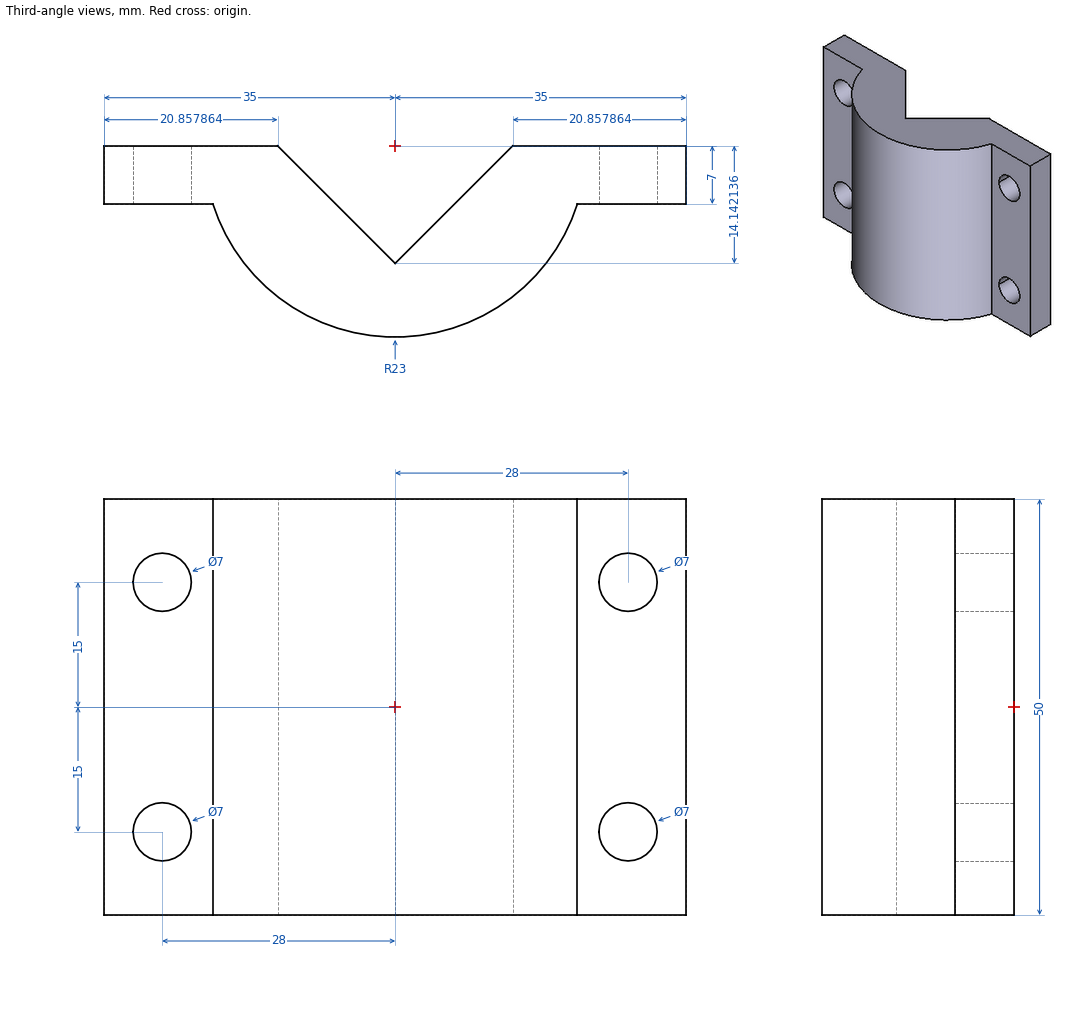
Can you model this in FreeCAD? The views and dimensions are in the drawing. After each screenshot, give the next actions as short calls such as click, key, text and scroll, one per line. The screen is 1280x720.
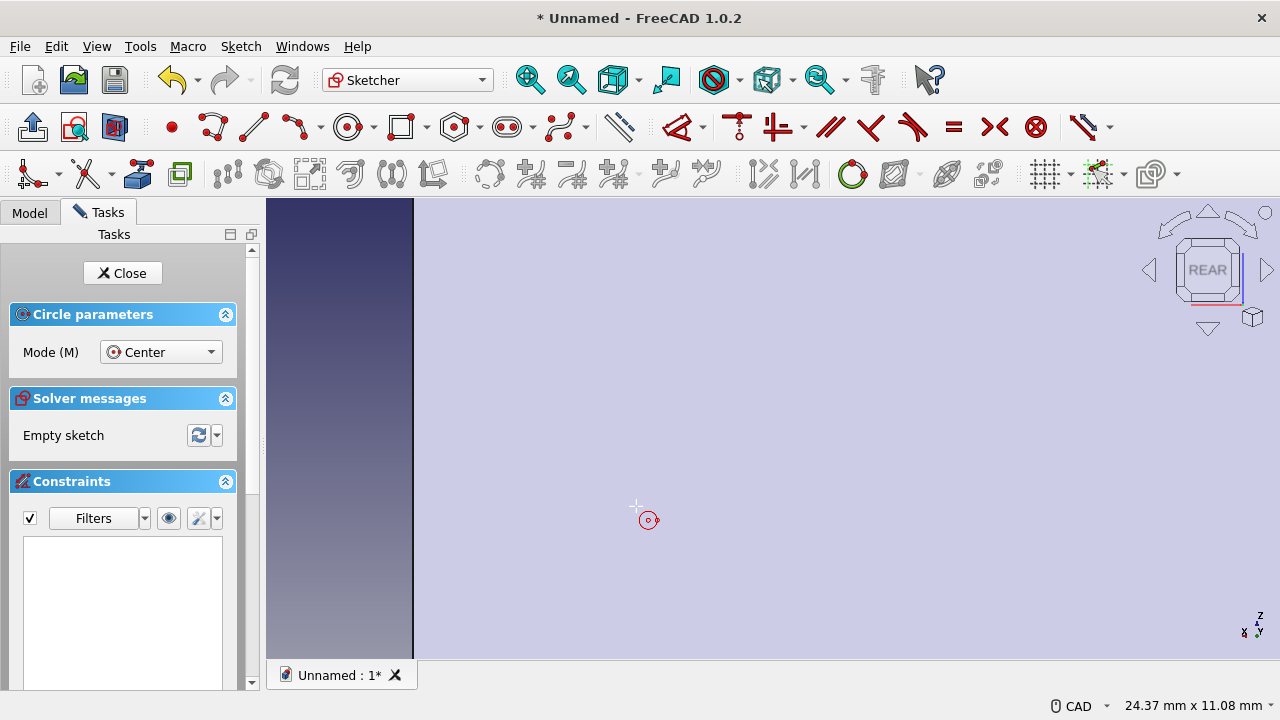
click(705, 425)
click(808, 322)
key(Escape)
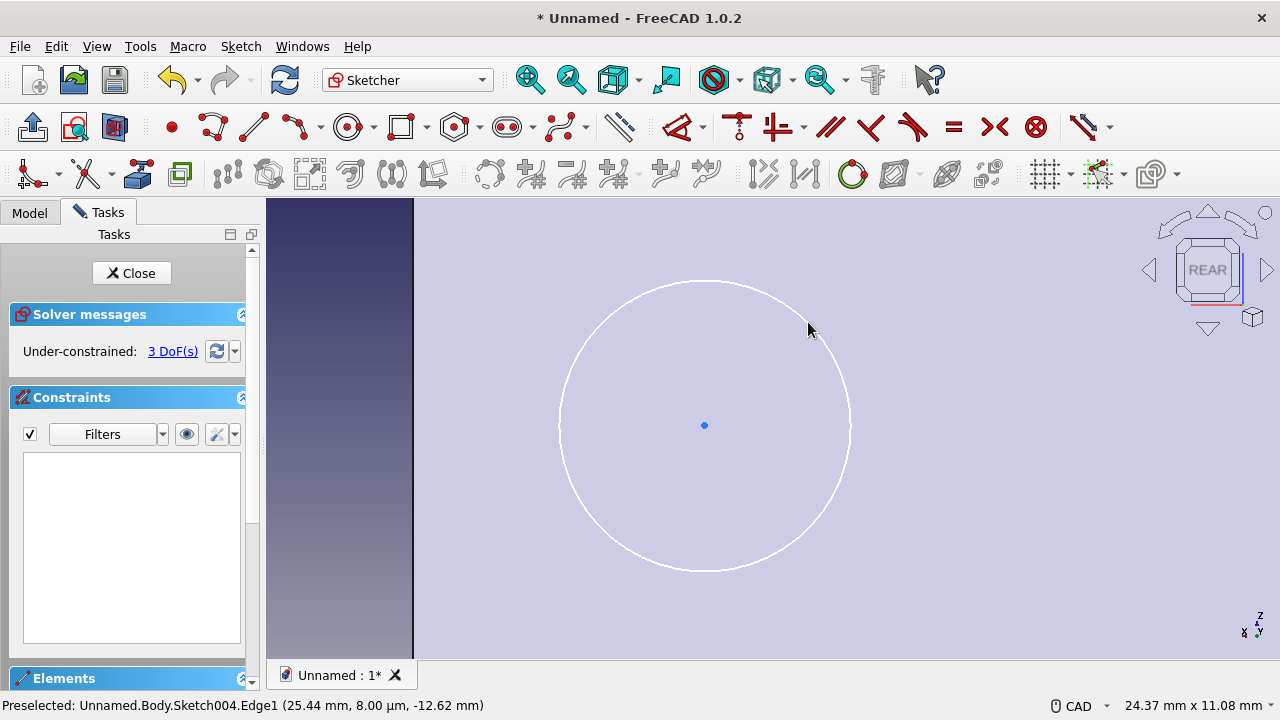
key(d)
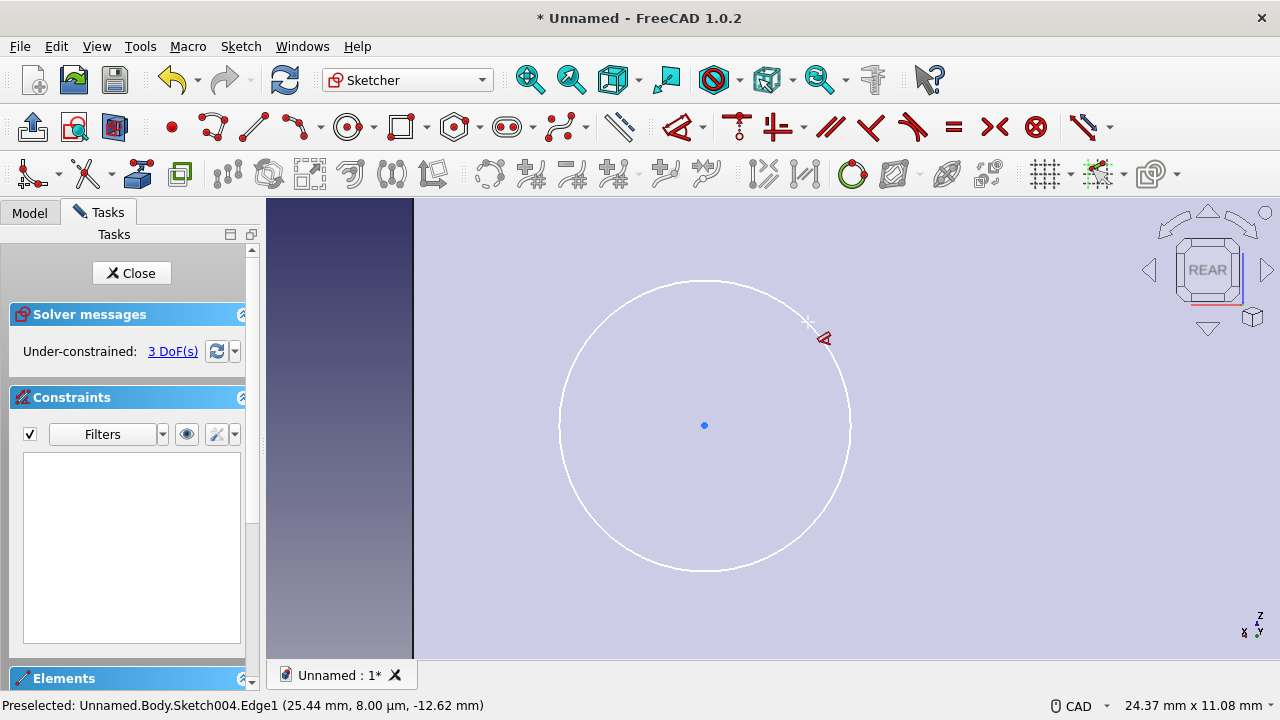
click(808, 323)
click(831, 300)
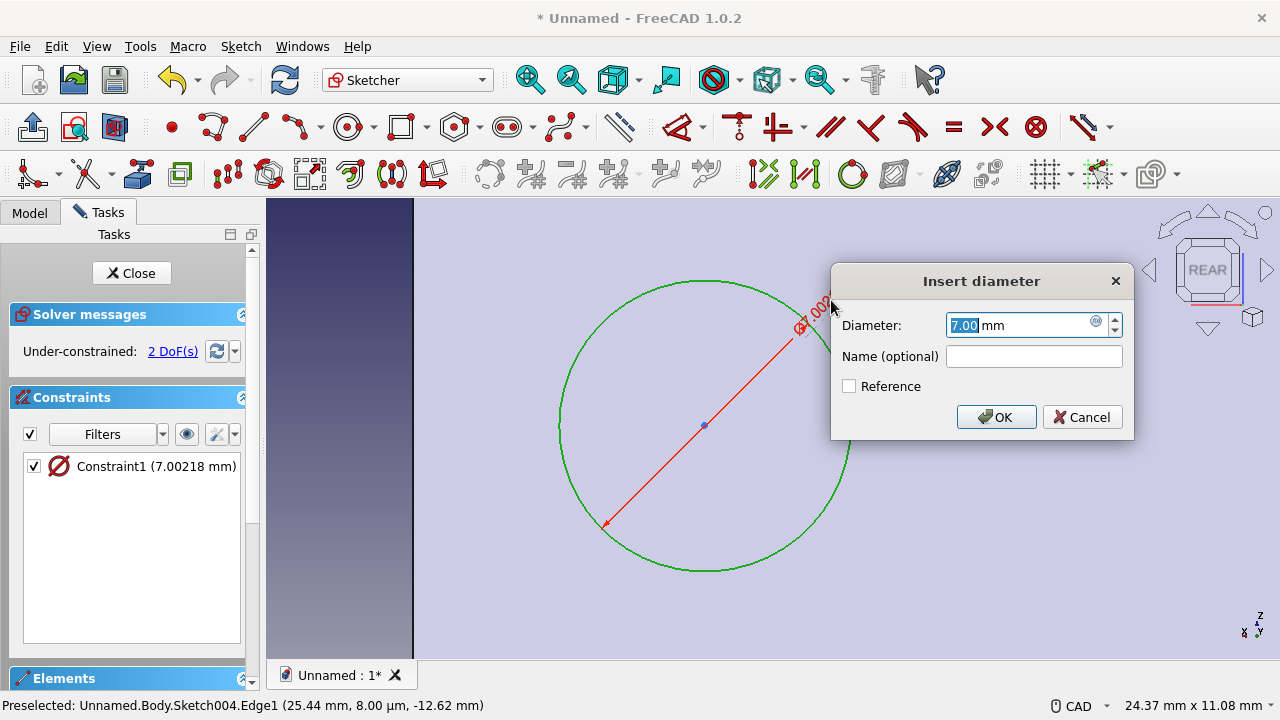
text(7)
key(Return)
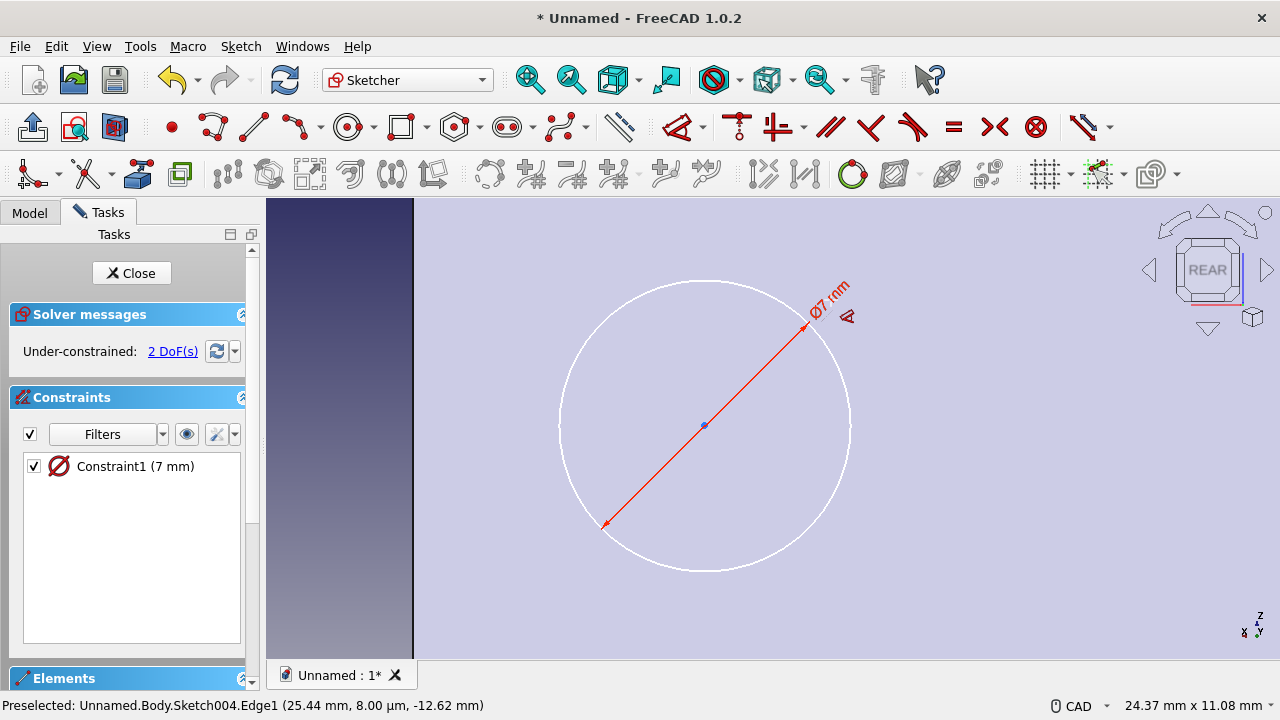
click(705, 426)
click(910, 460)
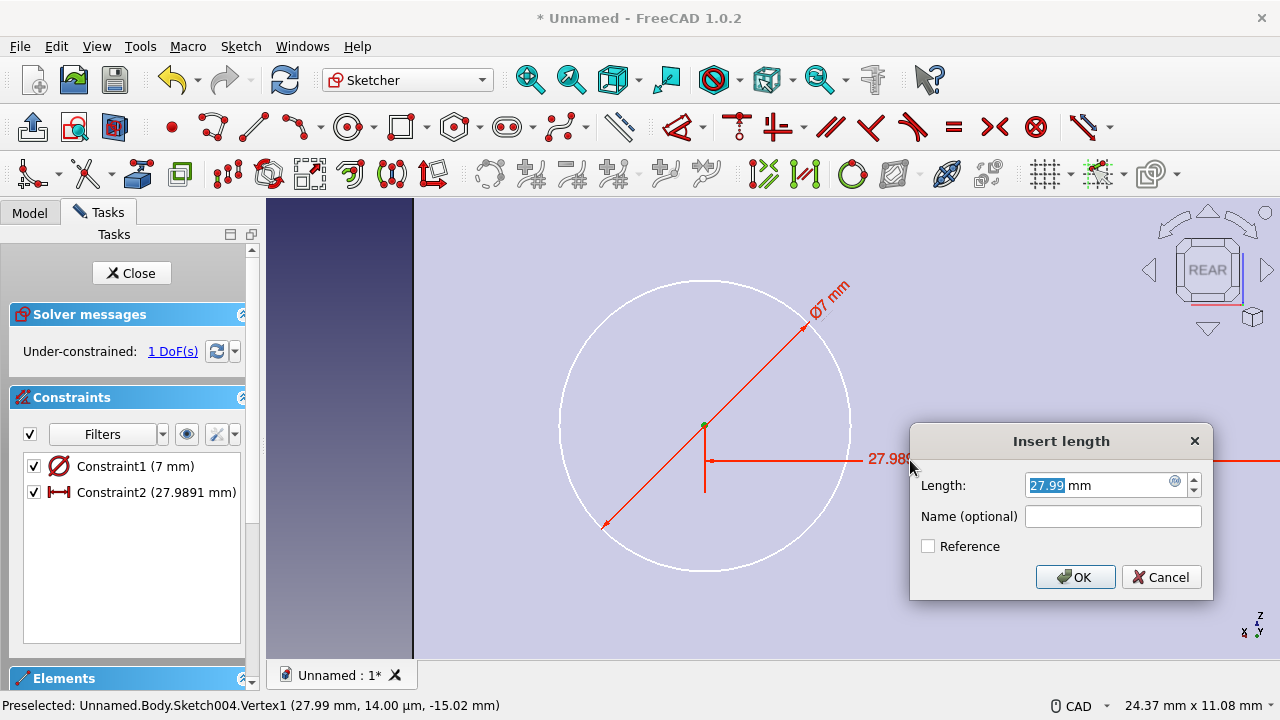
text(28)
key(Return)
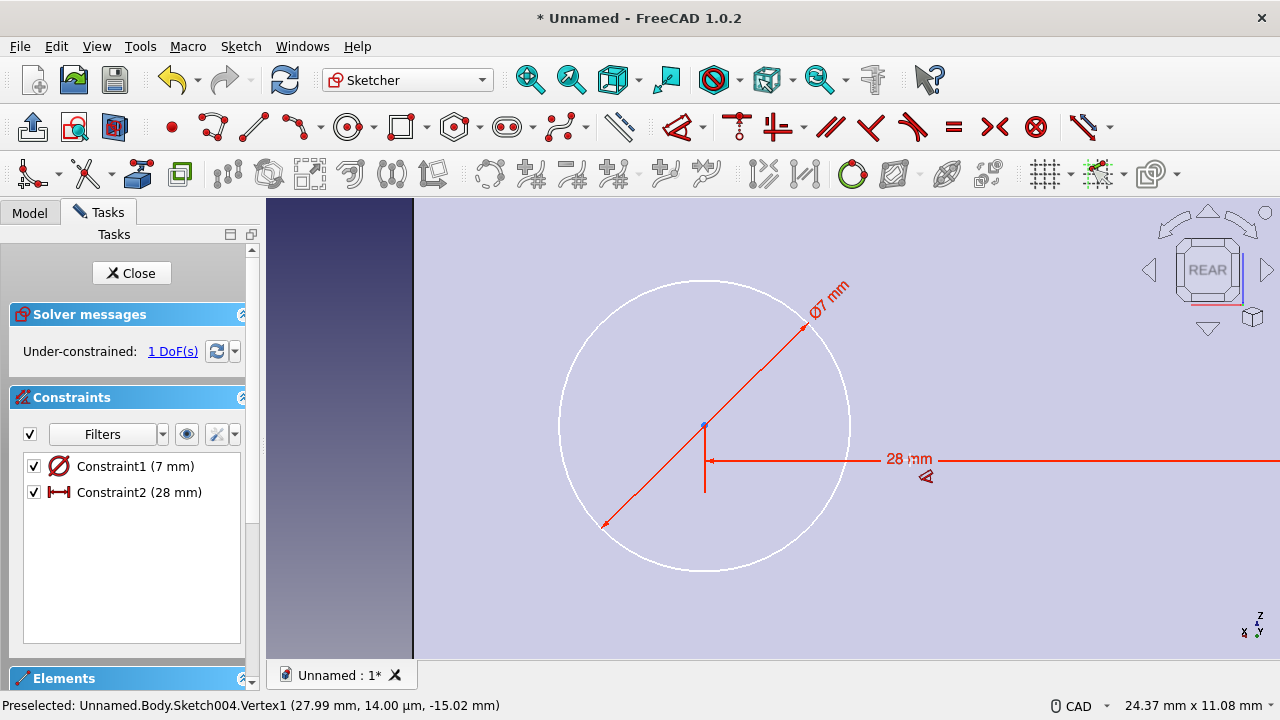
click(705, 426)
click(671, 326)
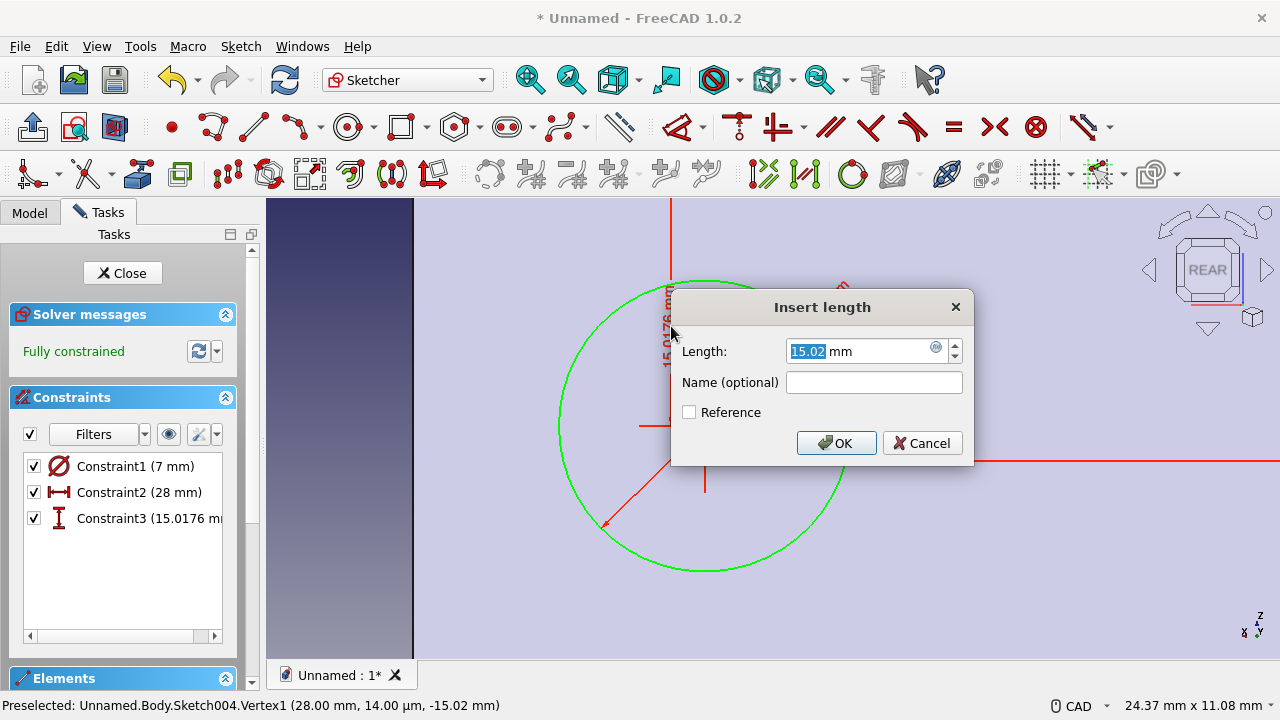
text(15)
key(Return)
key(Escape)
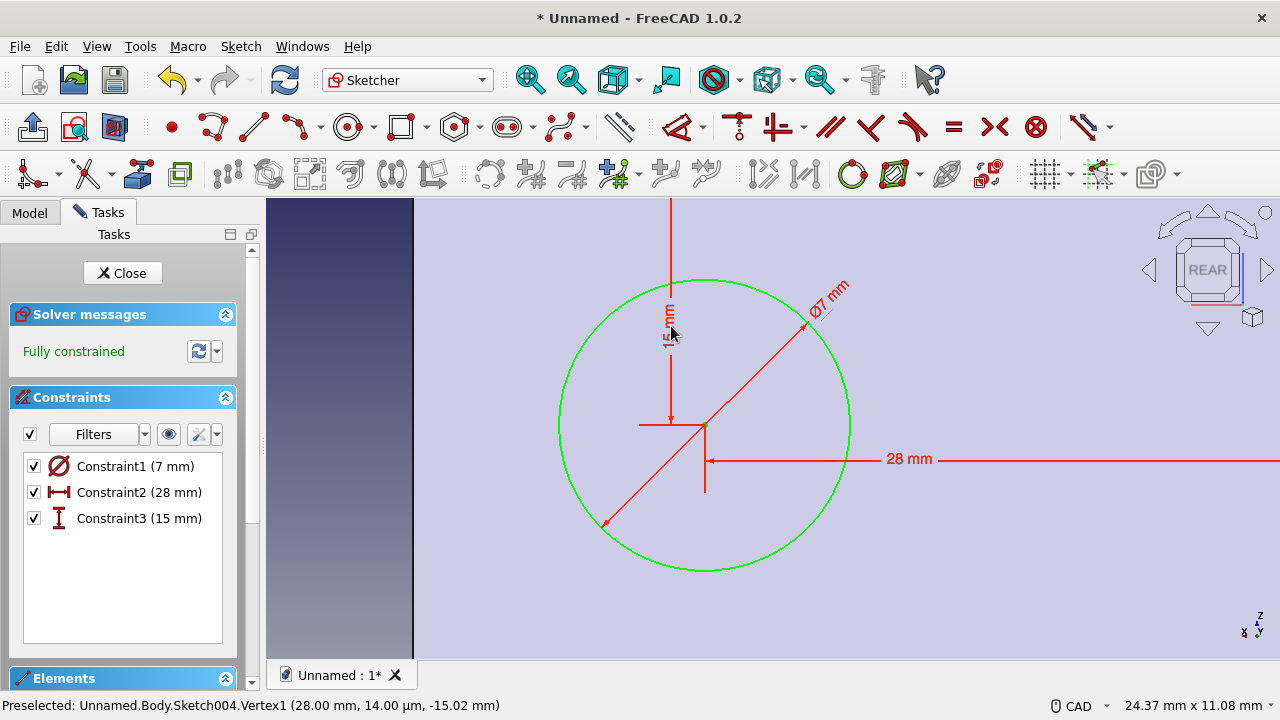
click(123, 273)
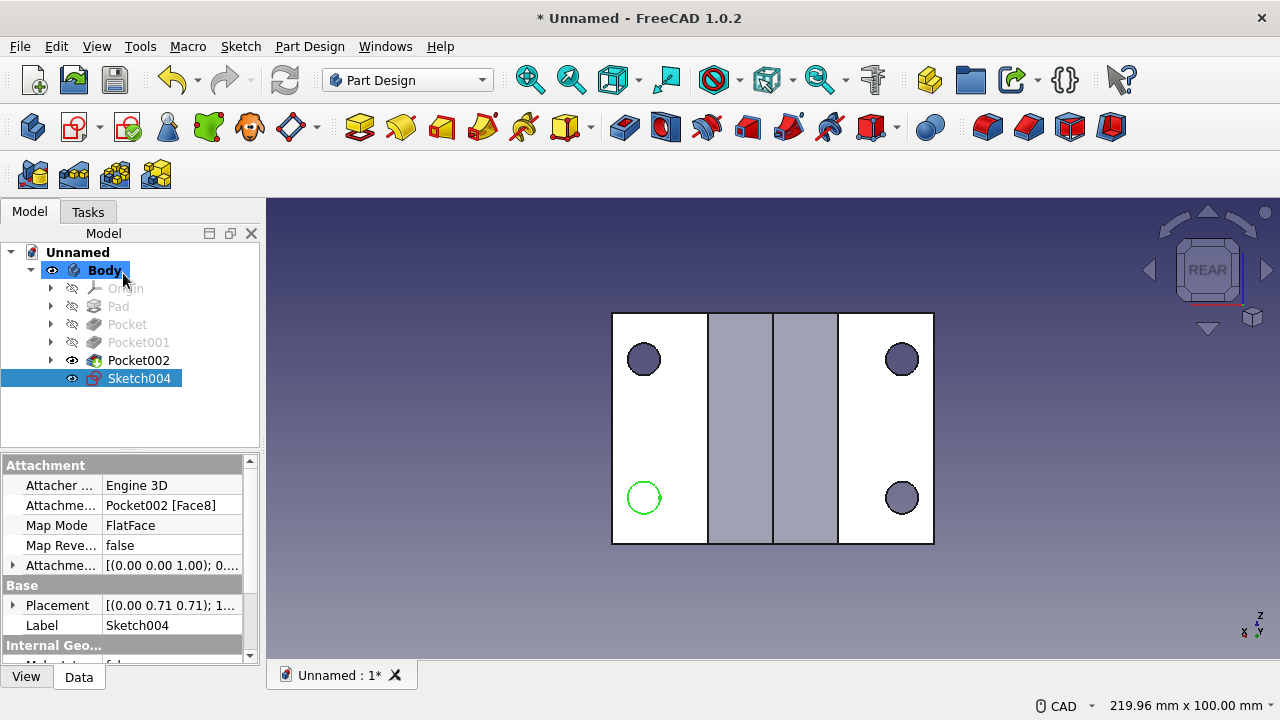
click(625, 128)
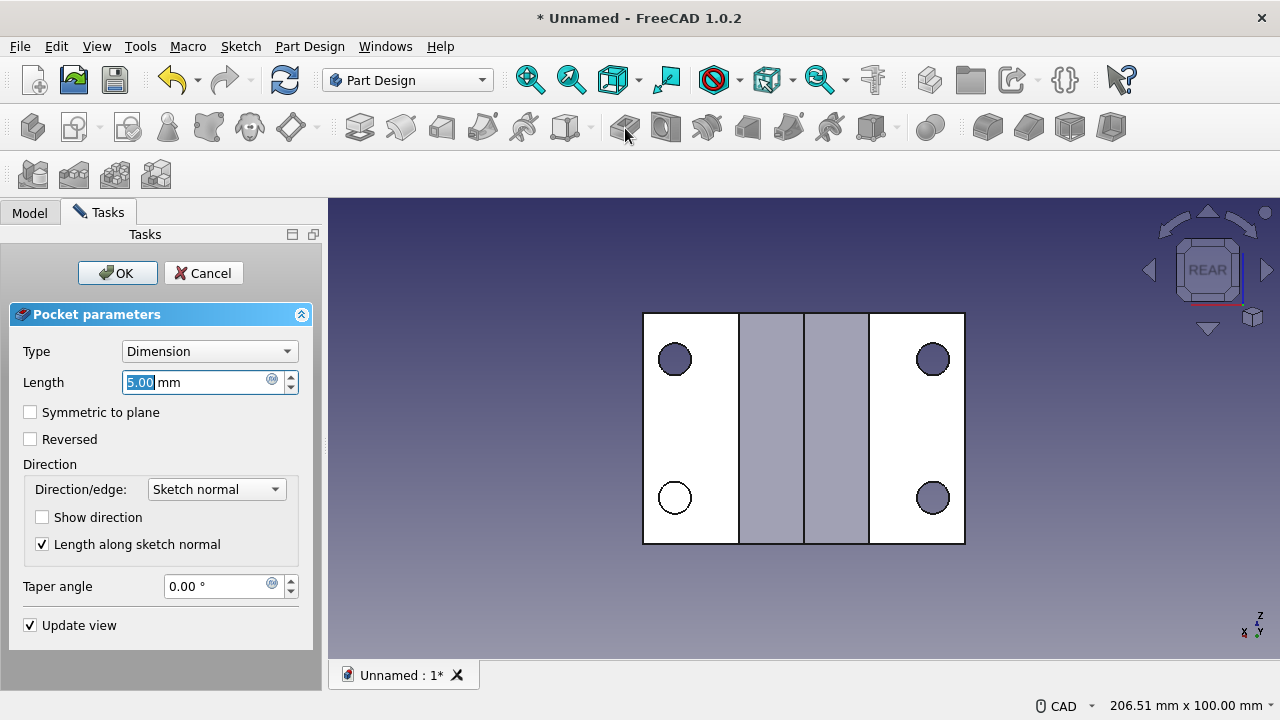
click(210, 352)